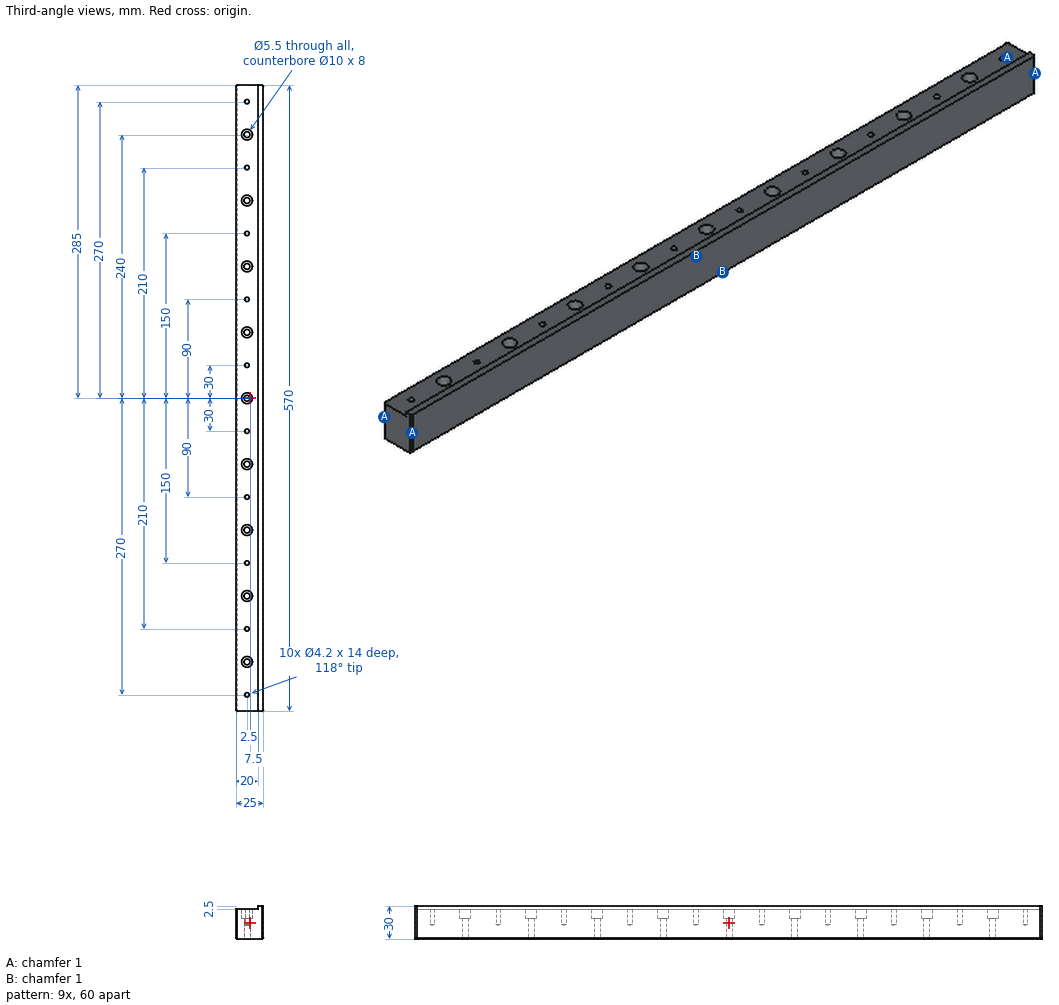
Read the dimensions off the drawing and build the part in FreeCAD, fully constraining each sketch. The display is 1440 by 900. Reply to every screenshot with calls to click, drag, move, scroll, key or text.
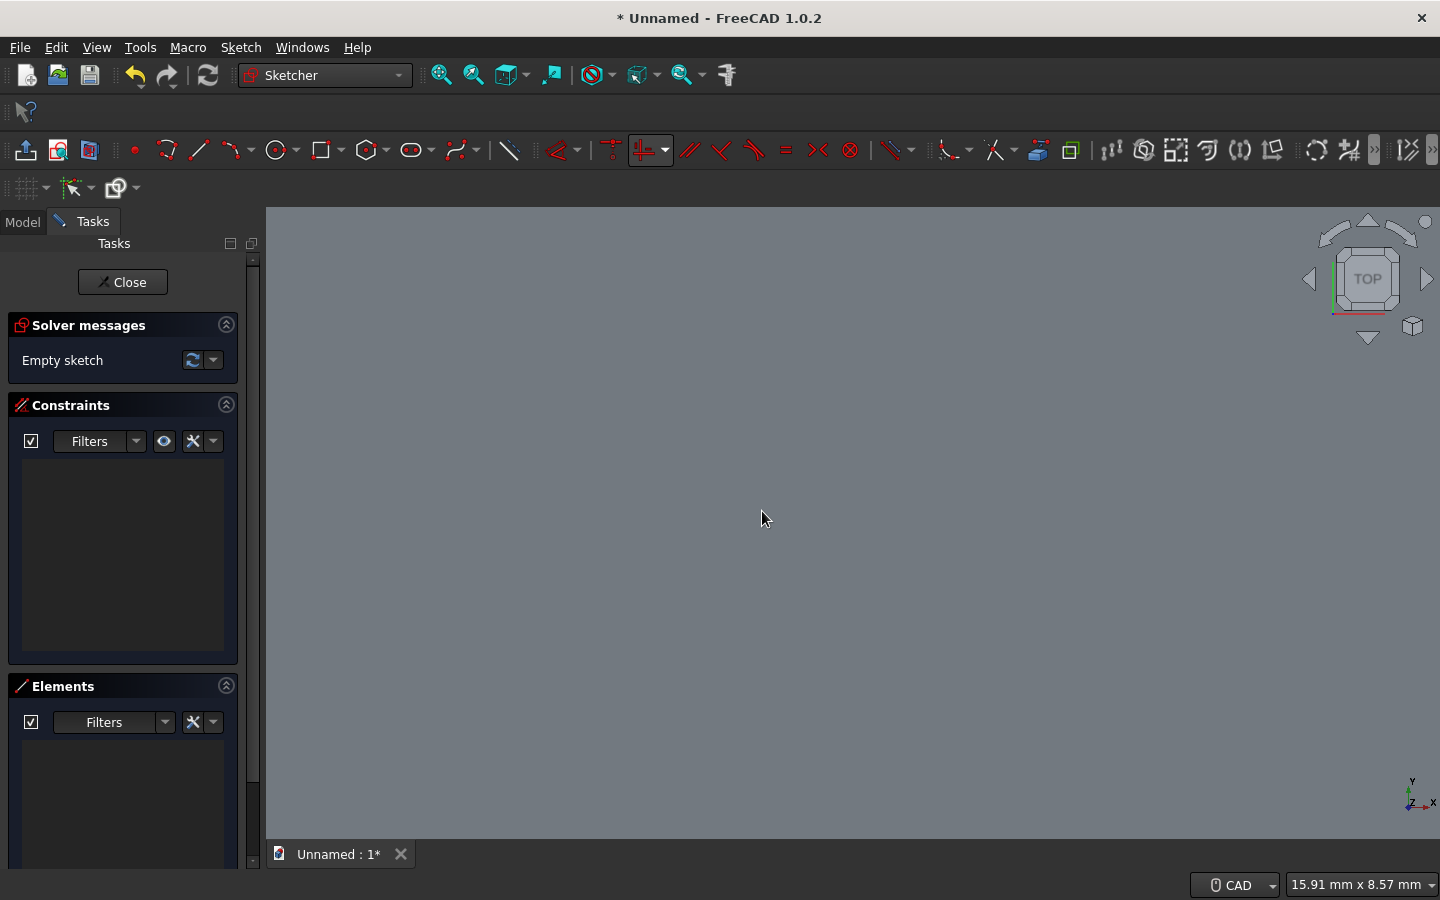
key(g)
key(c)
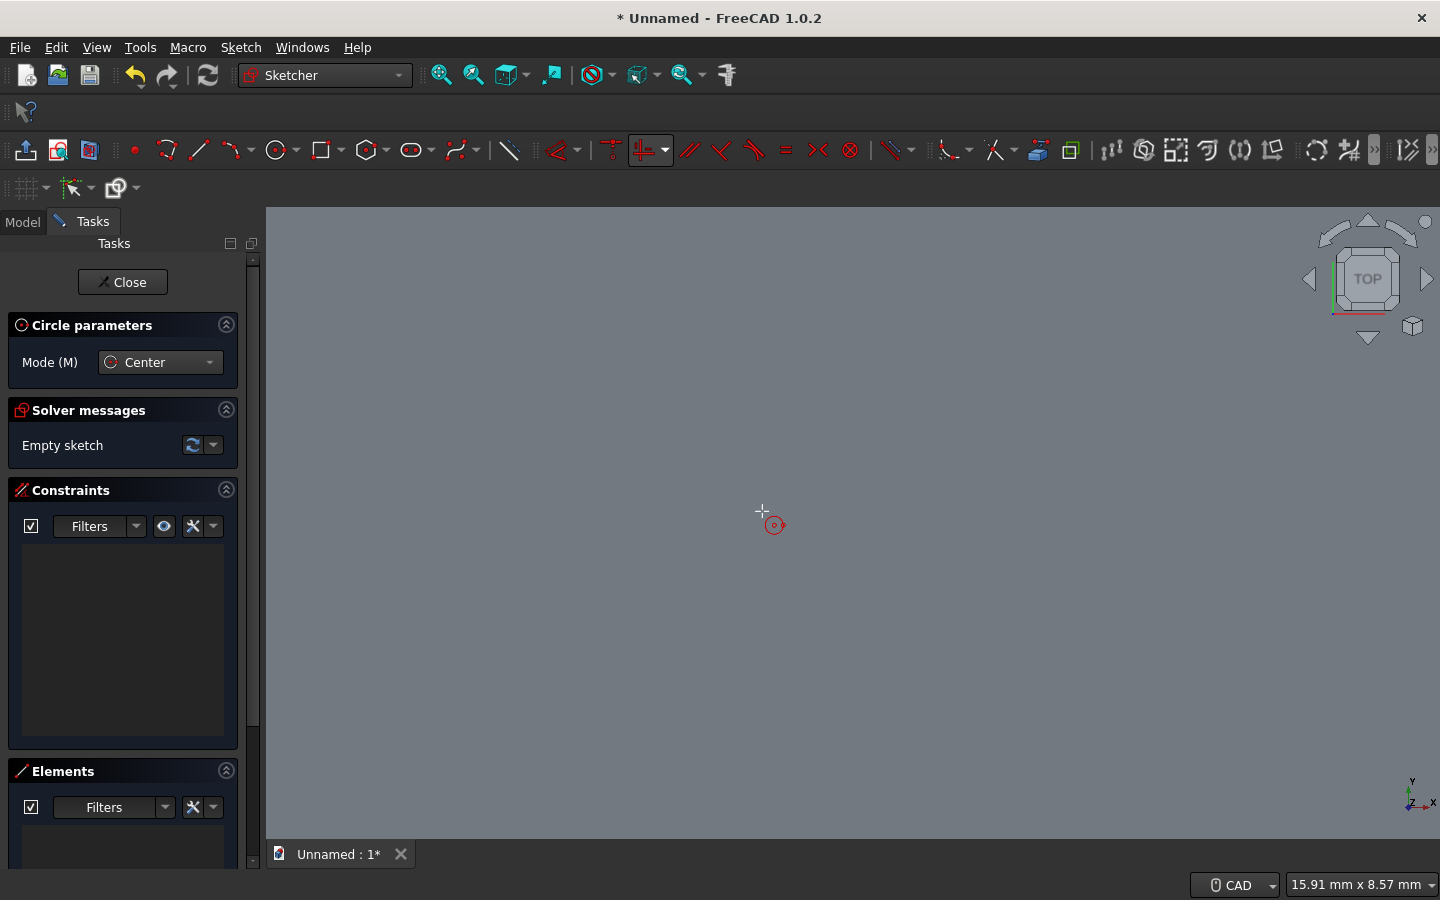
click(784, 521)
move(927, 378)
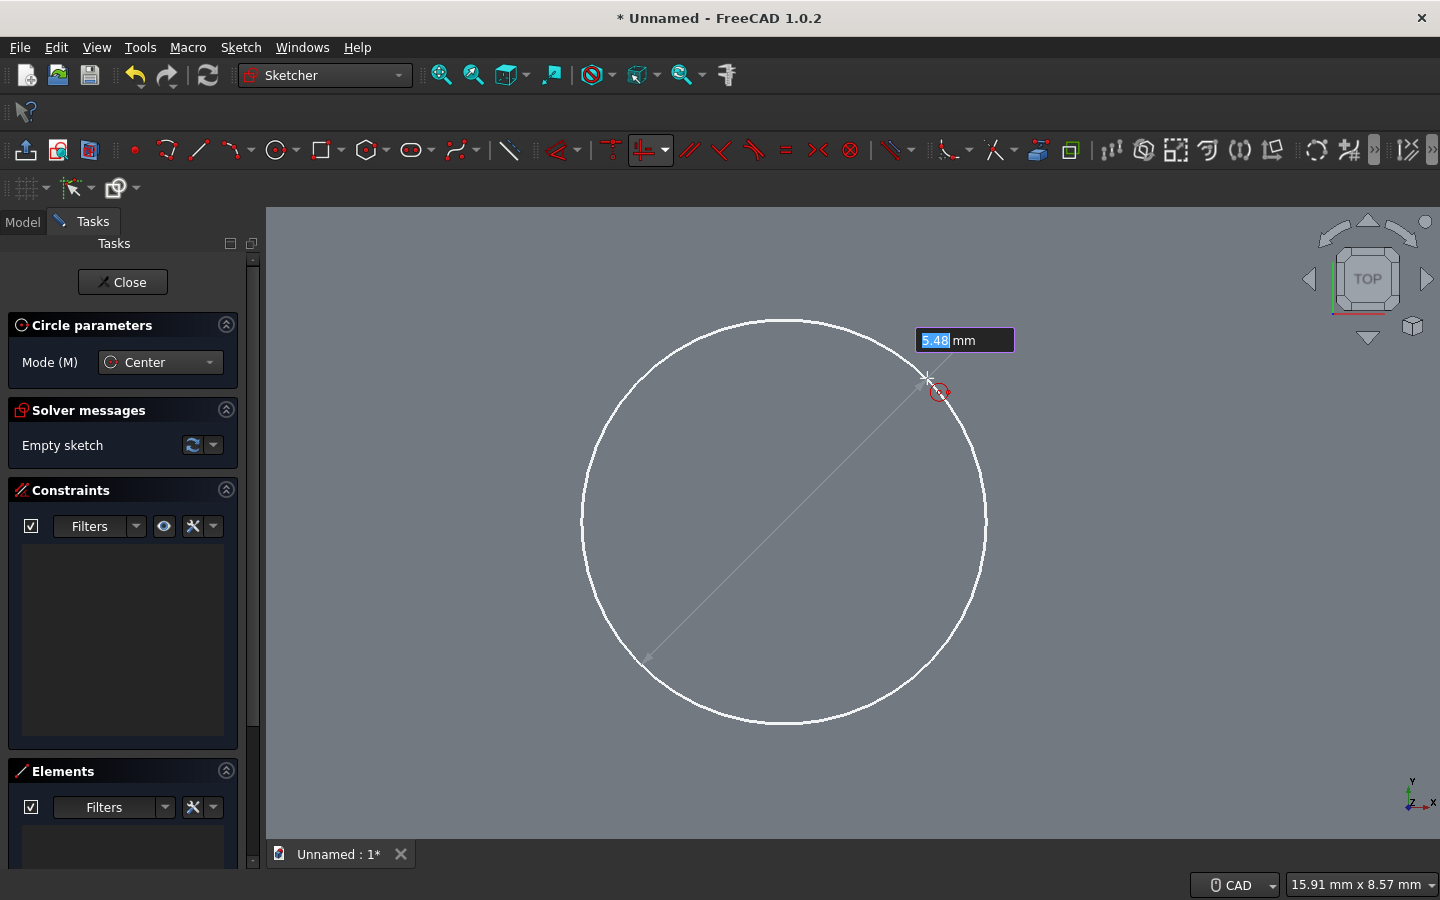
text(5.5)
key(Return)
key(Escape)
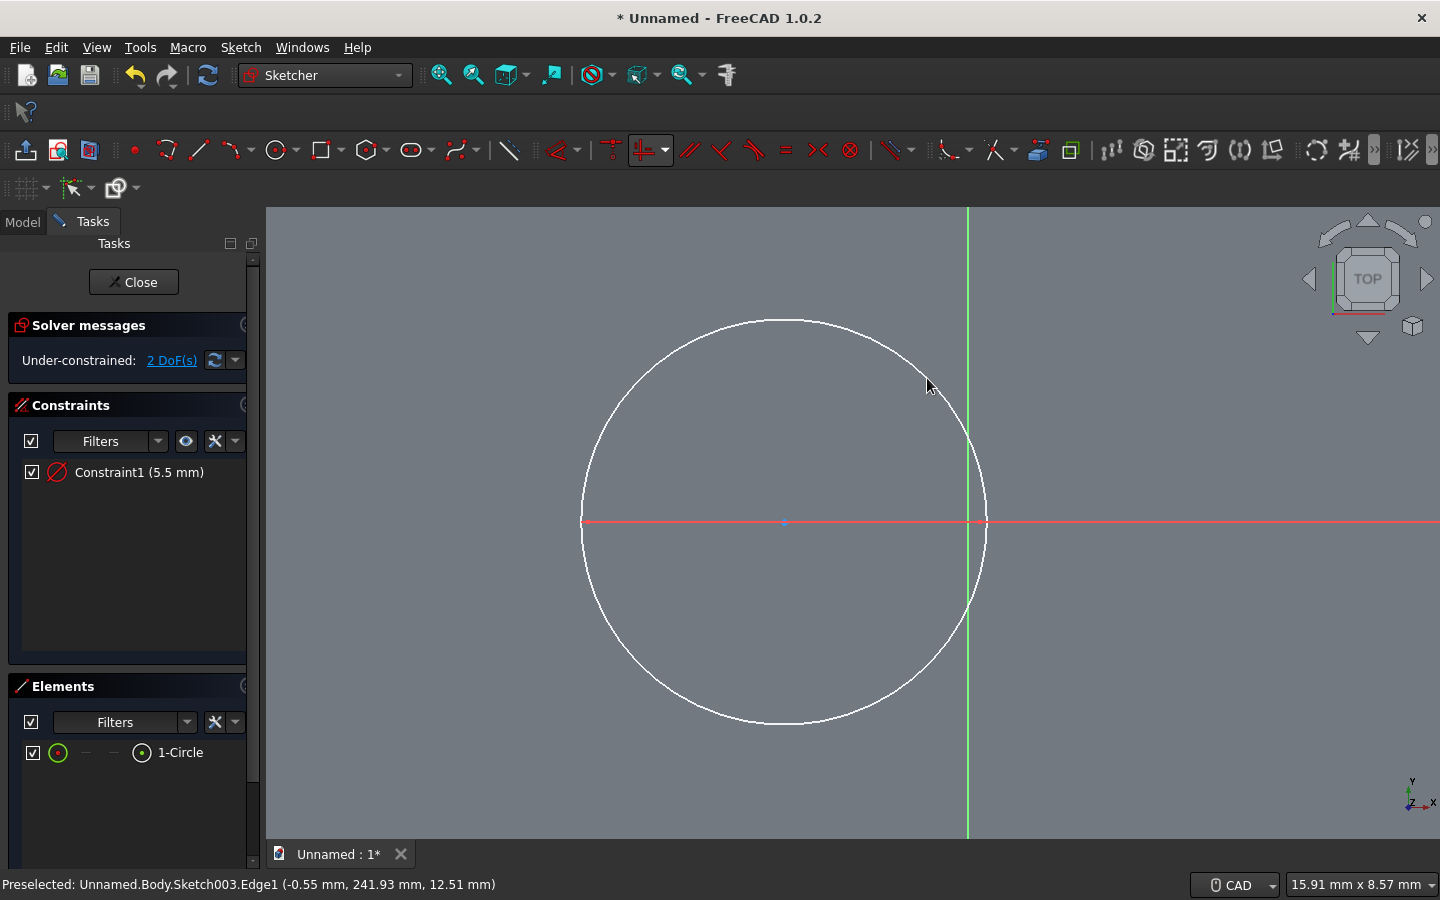
click(556, 150)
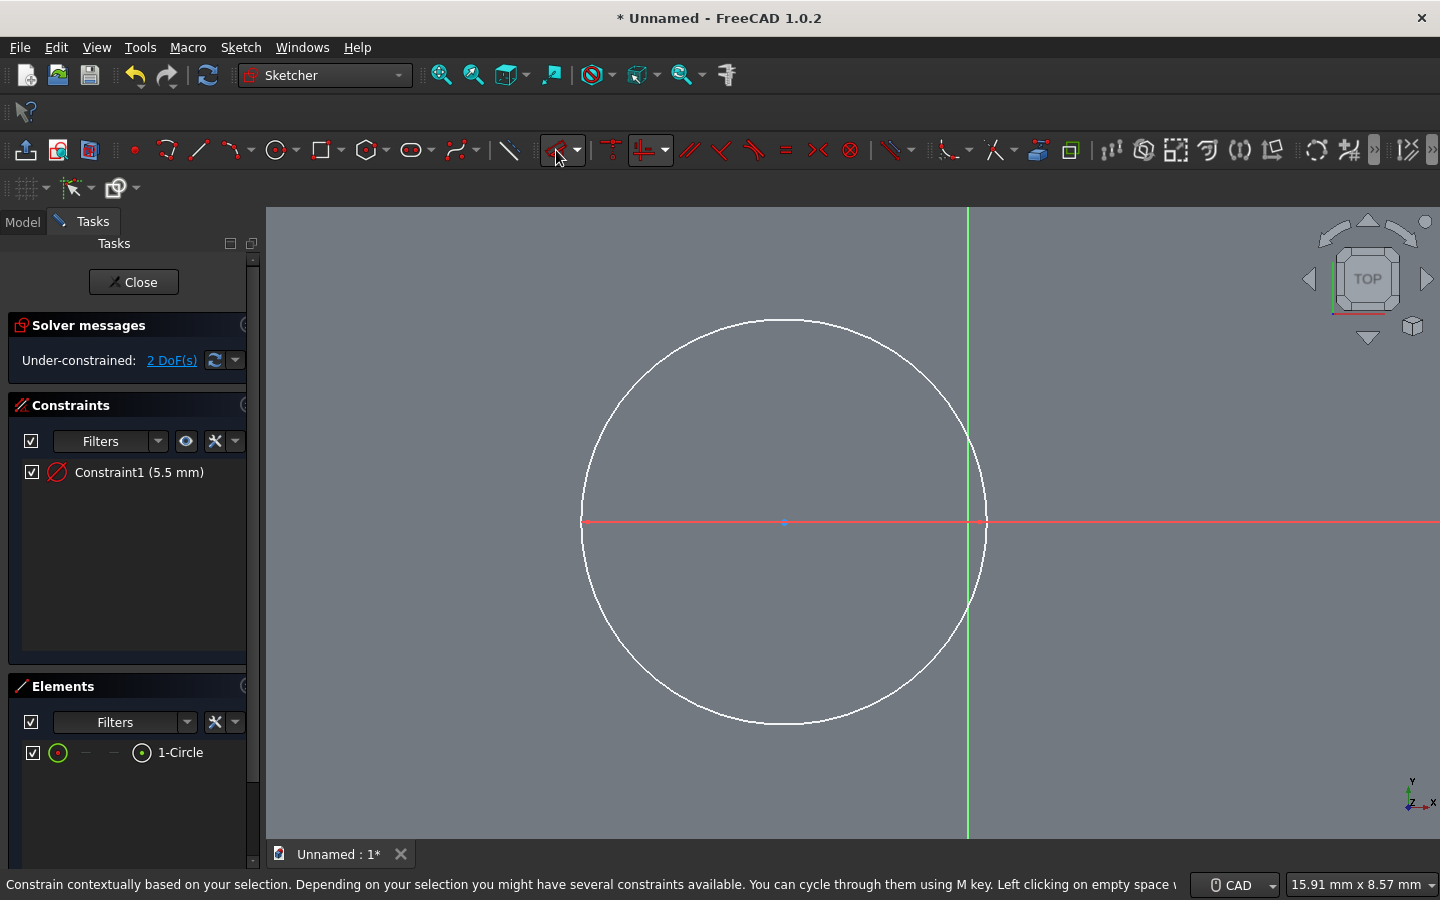
click(784, 522)
click(876, 488)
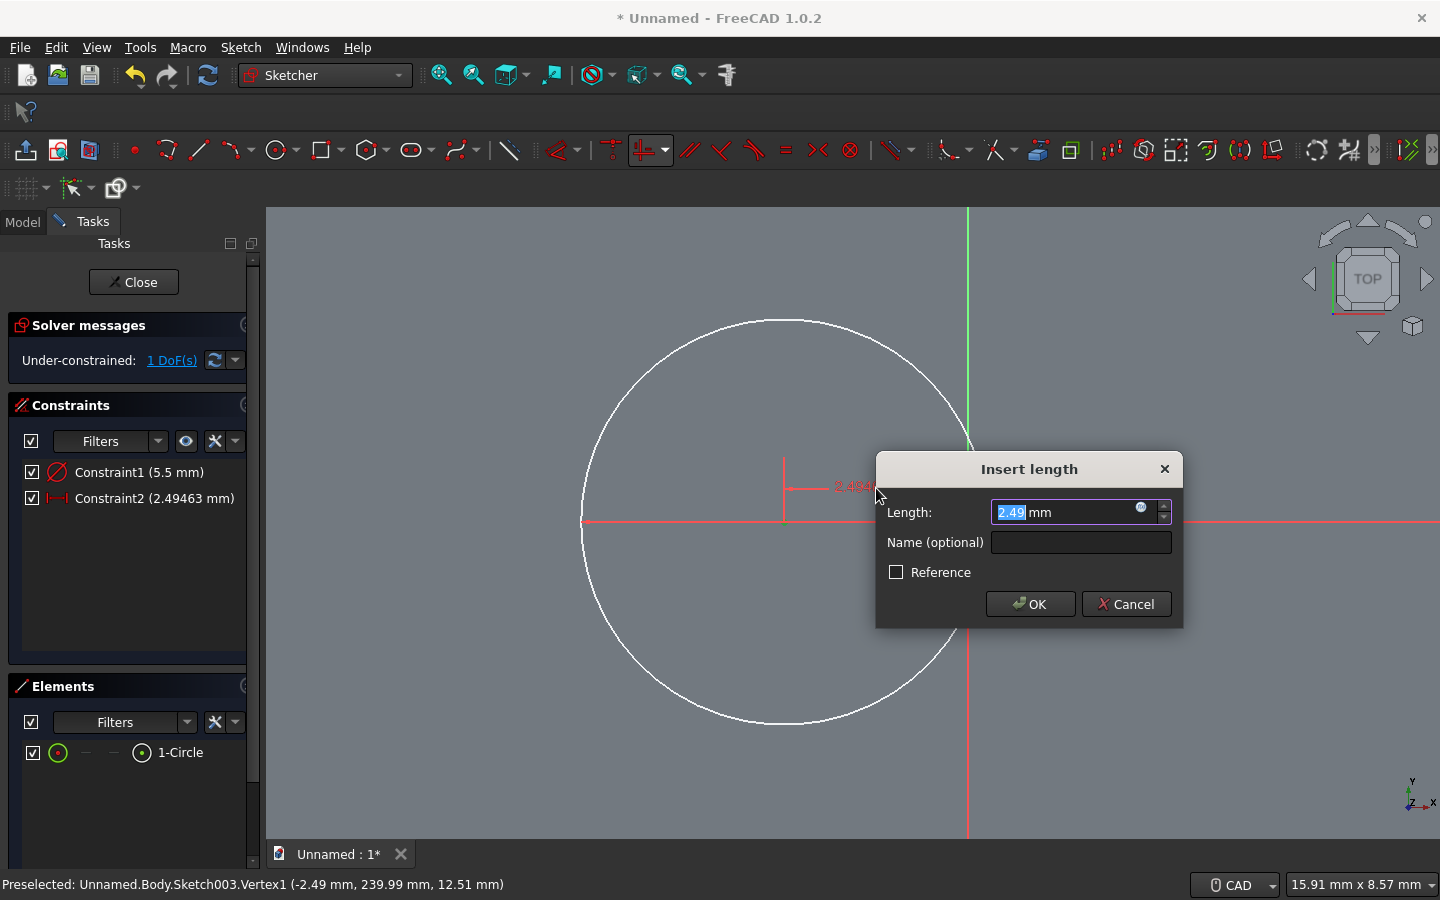
text(2.5)
key(Return)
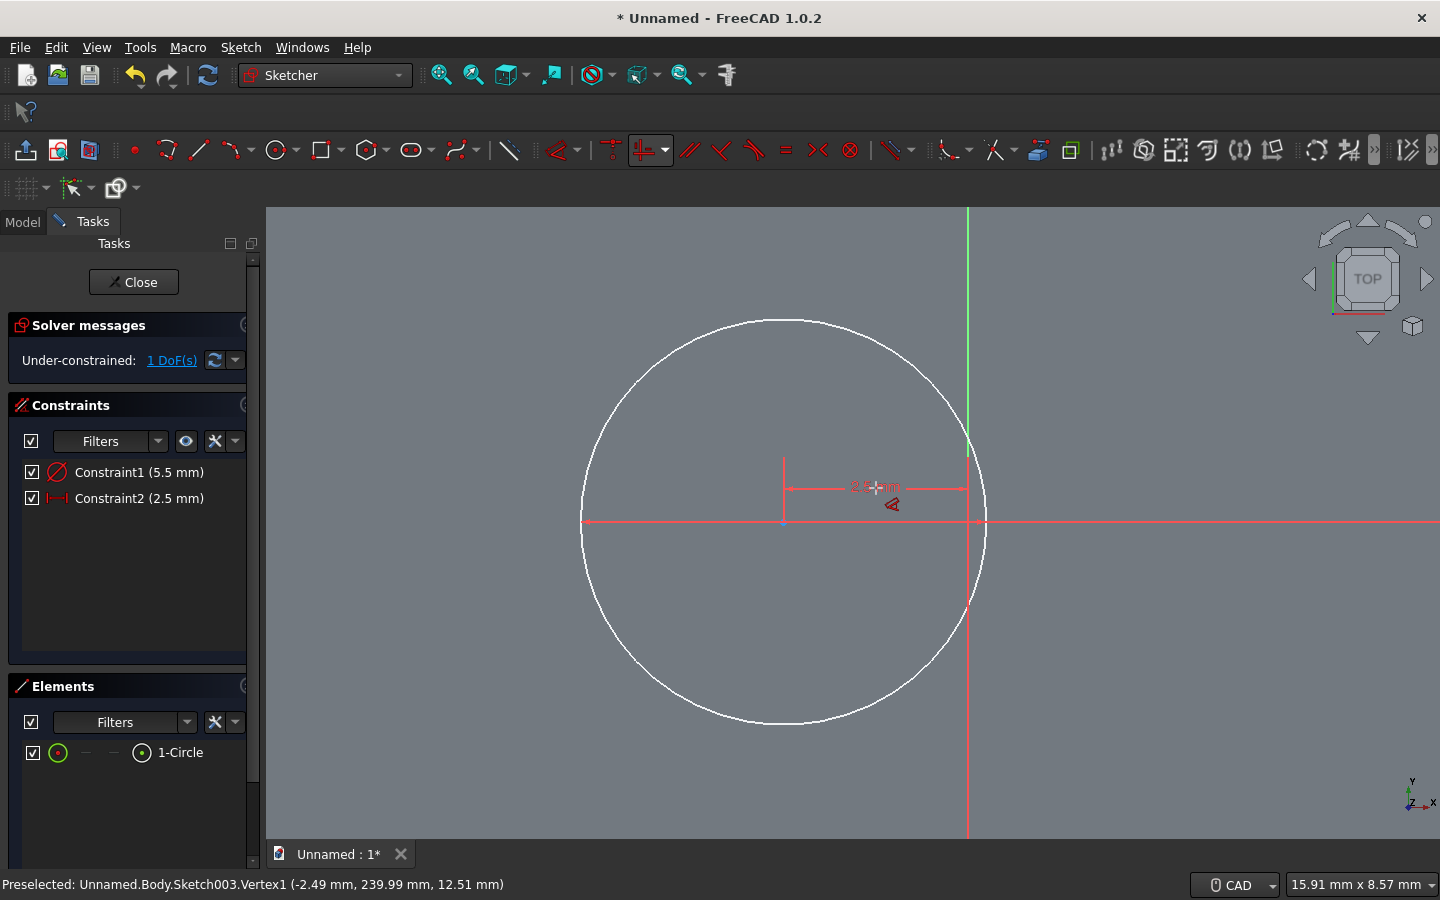
click(784, 522)
click(1002, 667)